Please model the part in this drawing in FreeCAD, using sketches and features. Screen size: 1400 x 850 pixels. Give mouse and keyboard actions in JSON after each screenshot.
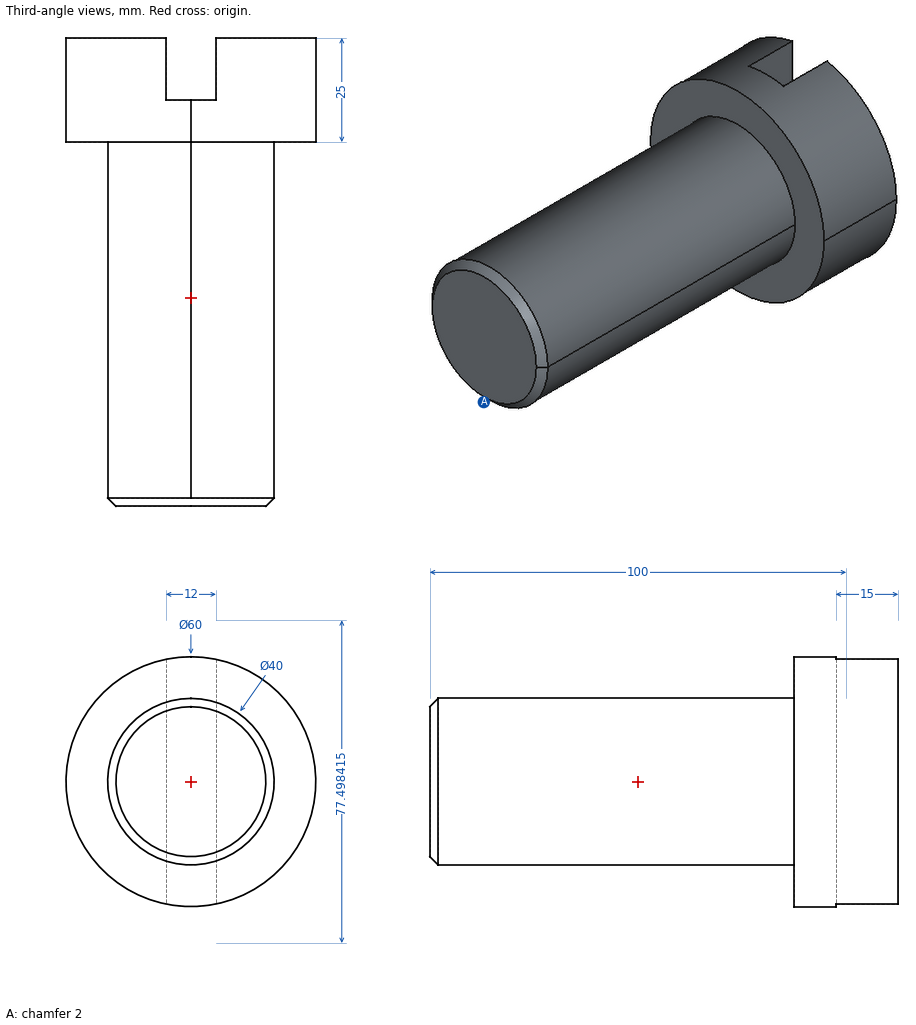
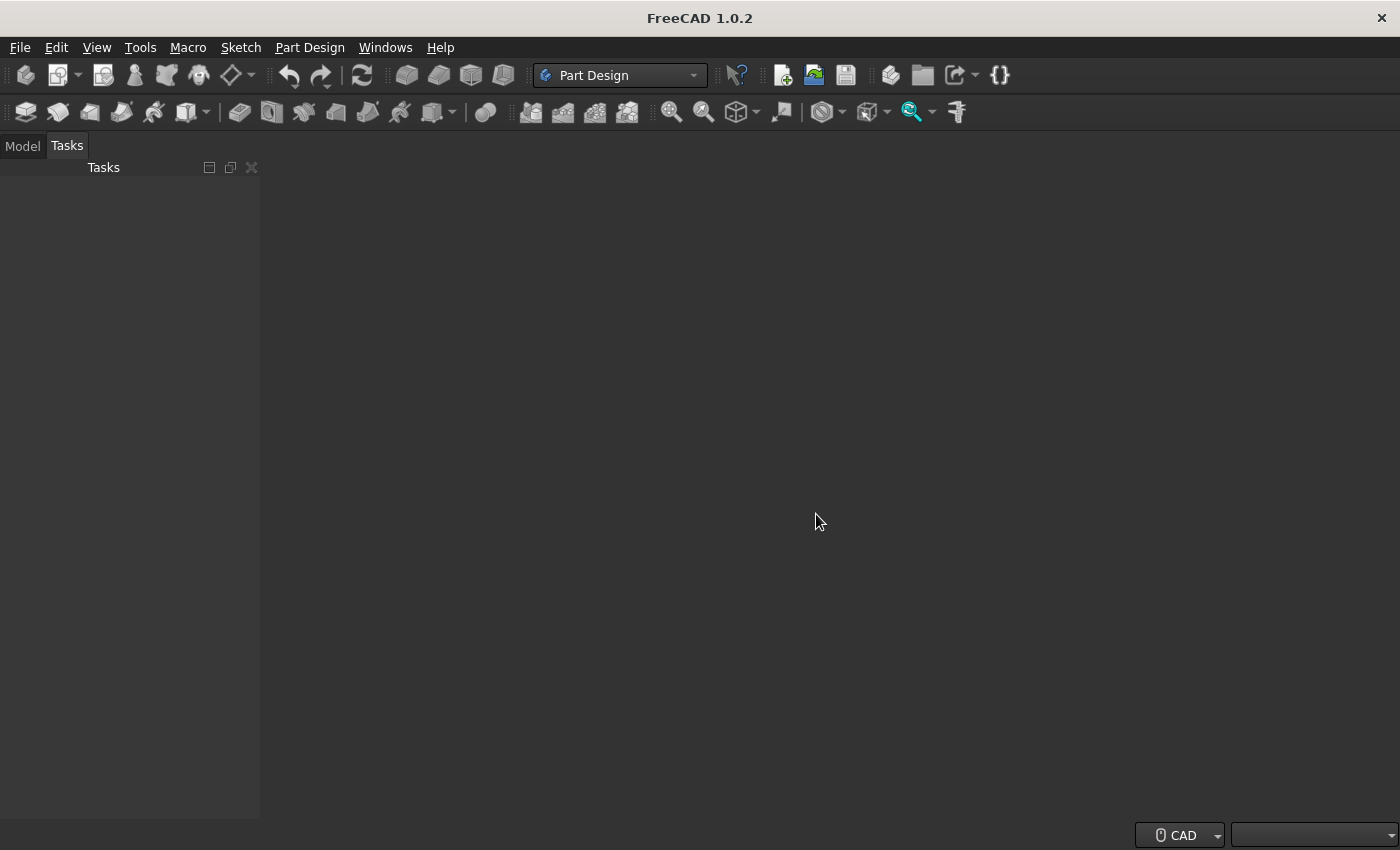
{"action": "left_click", "coordinate": [782, 76]}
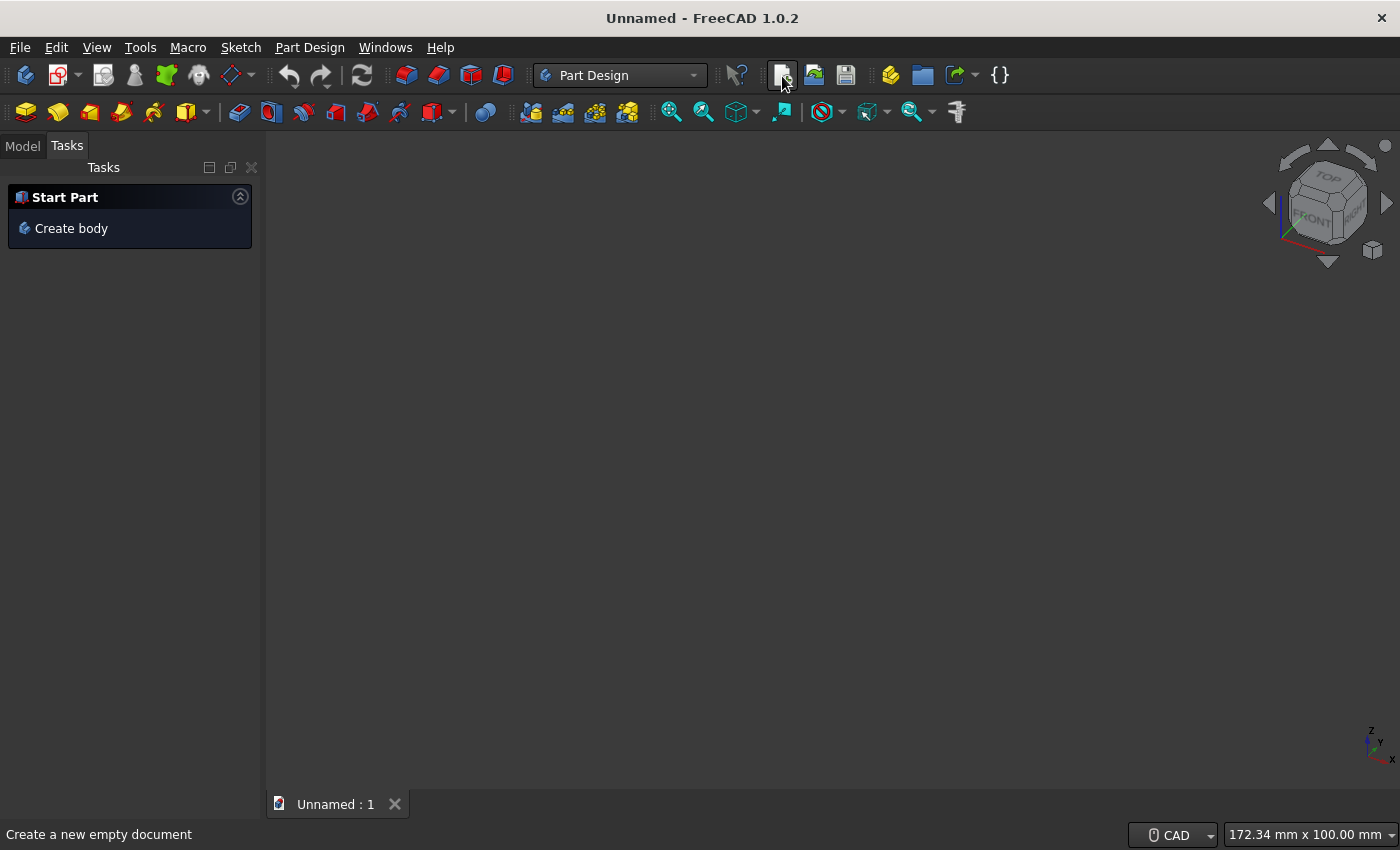
{"action": "left_click", "coordinate": [58, 76]}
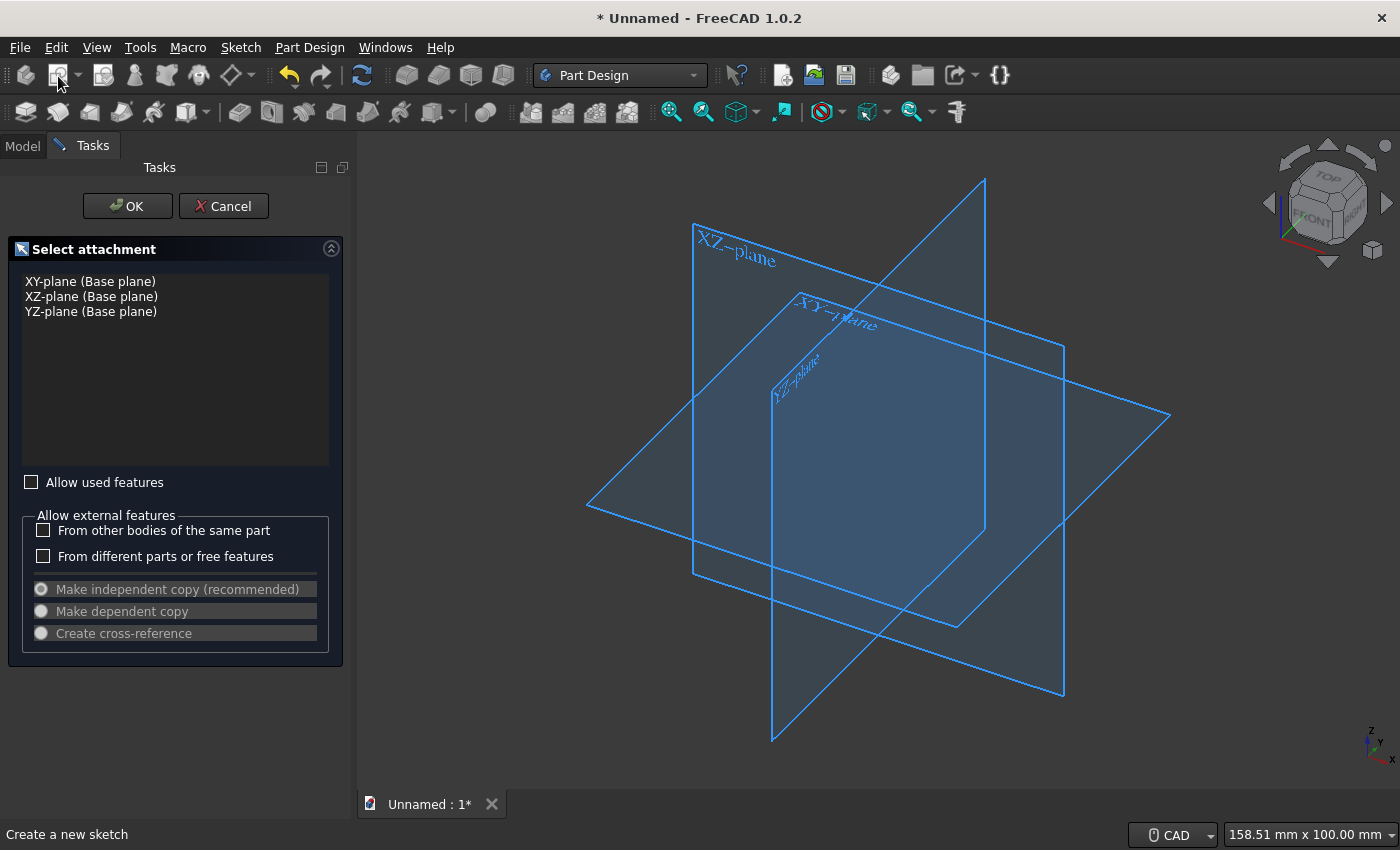
{"action": "left_click", "coordinate": [82, 296]}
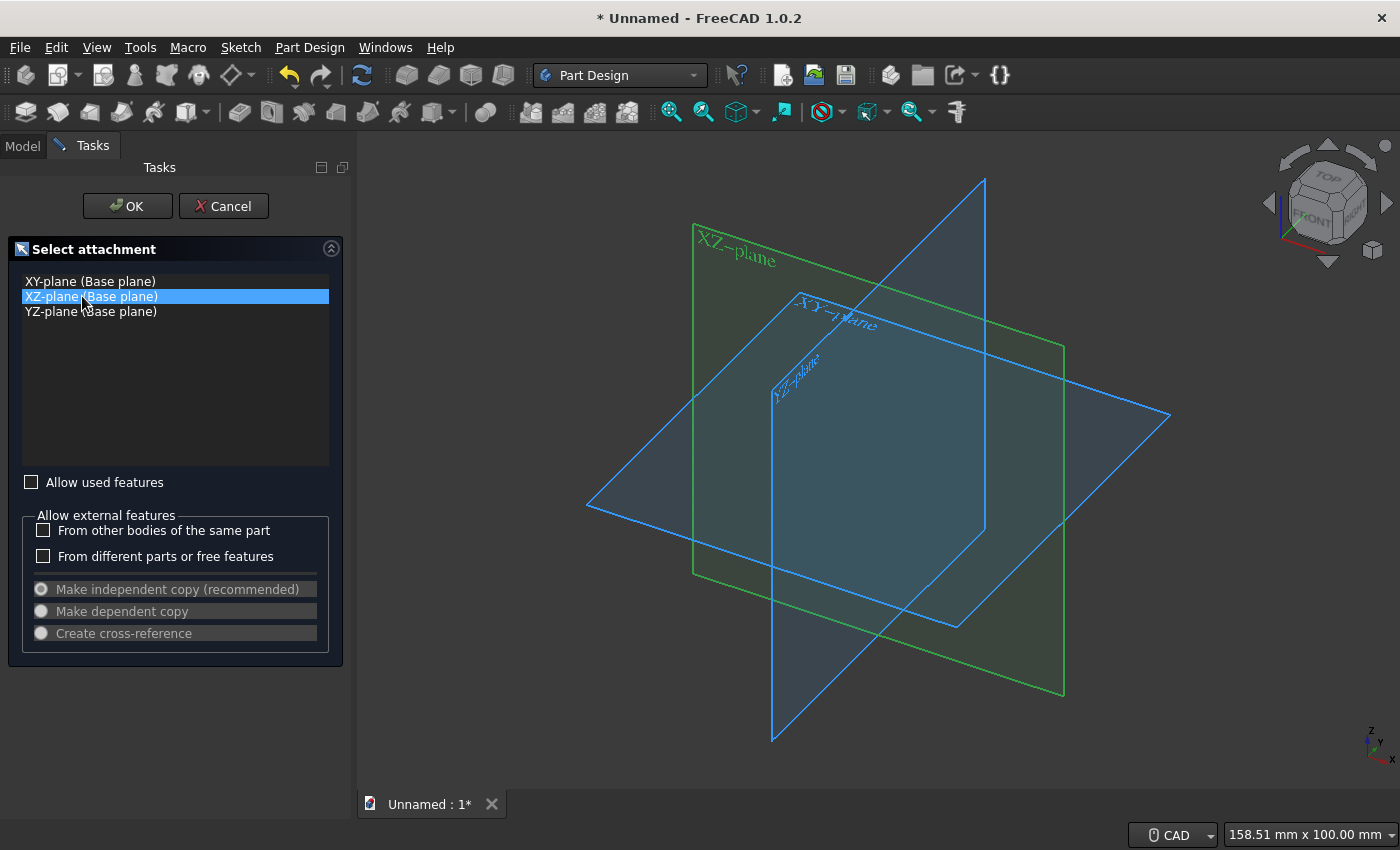
{"action": "left_click", "coordinate": [128, 206]}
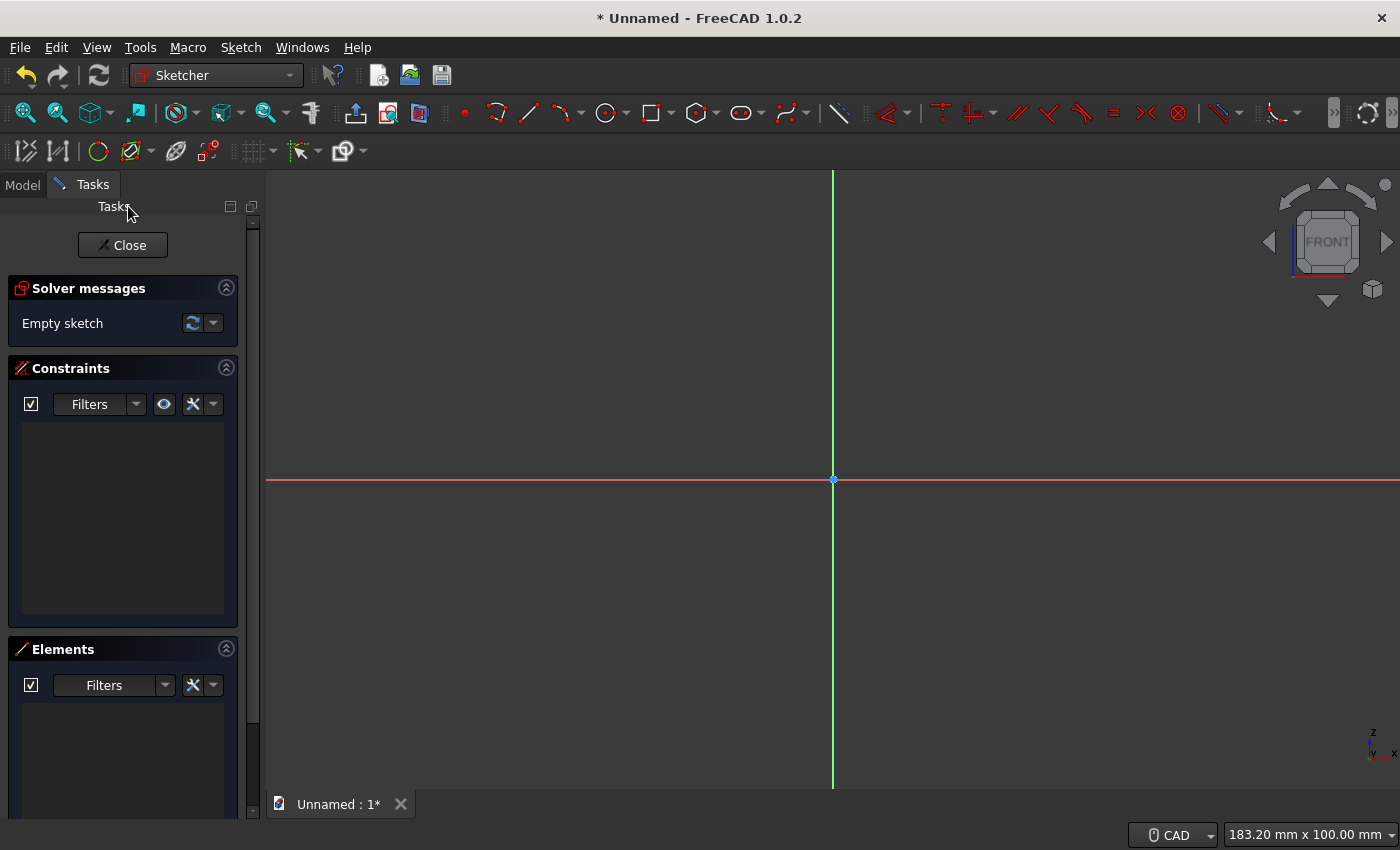
{"action": "scroll", "coordinate": [972, 480], "scroll_direction": "up", "scroll_amount": 2}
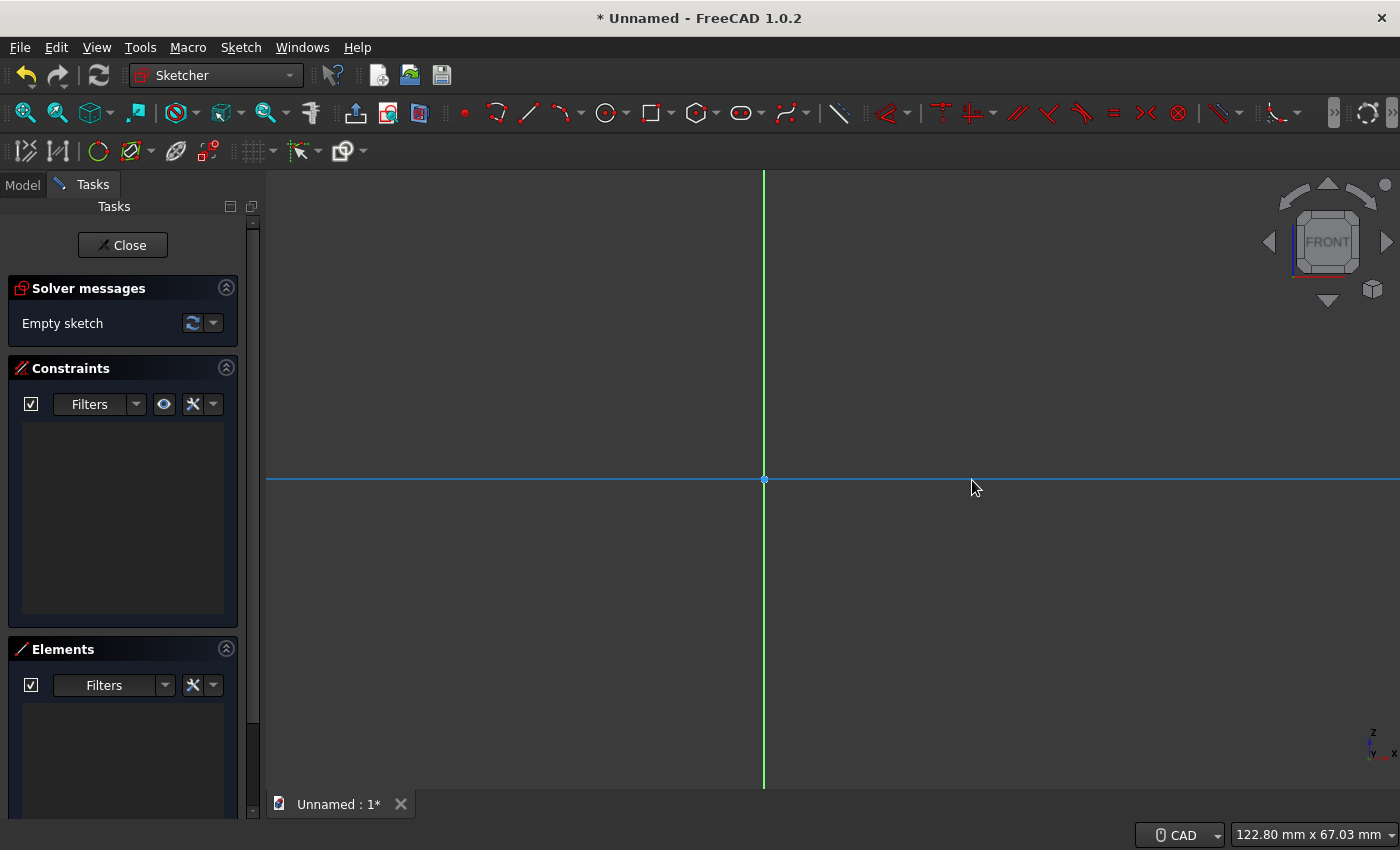
{"action": "left_click", "coordinate": [606, 114]}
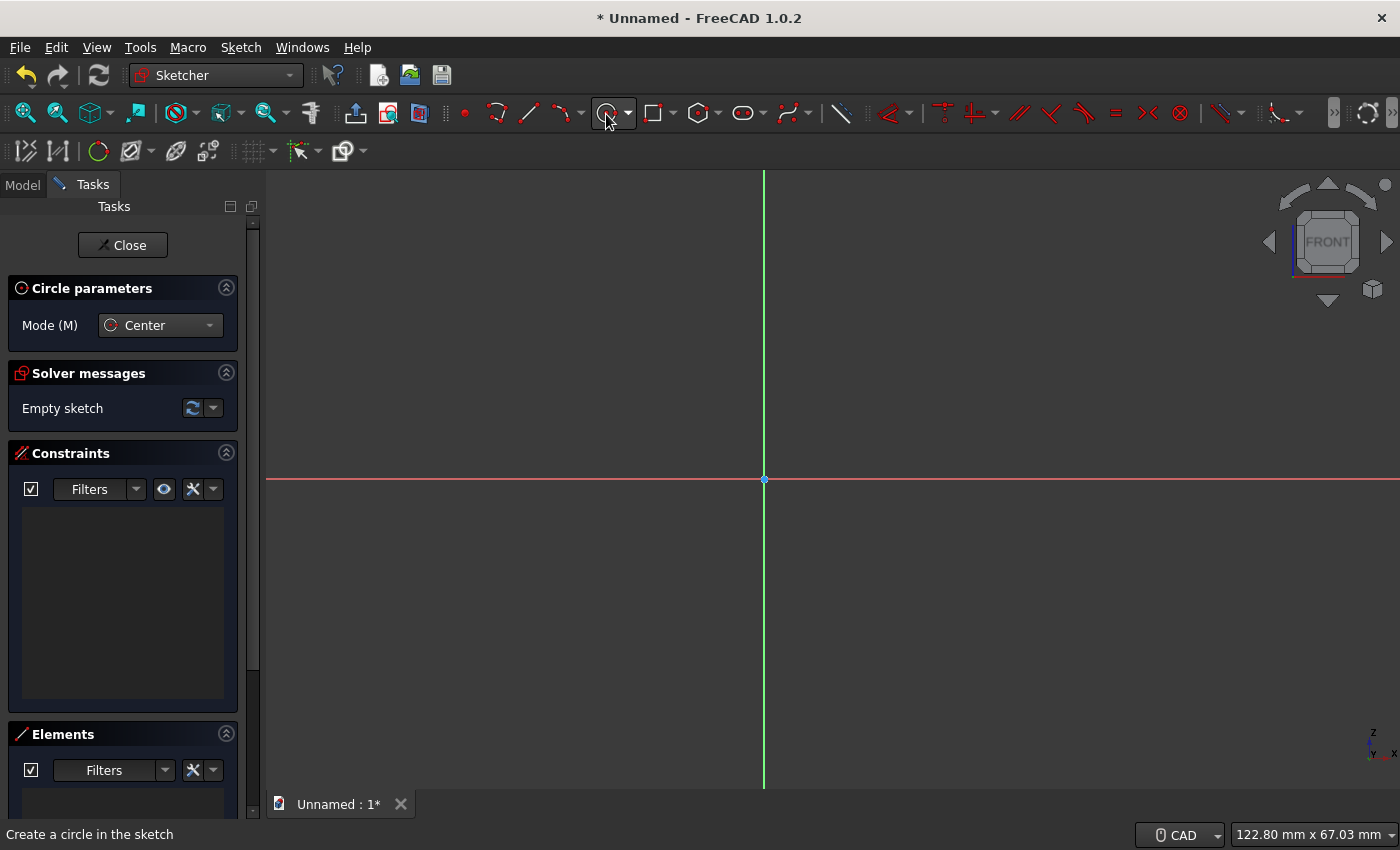
{"action": "left_click", "coordinate": [764, 479]}
{"action": "mouse_move", "coordinate": [895, 348]}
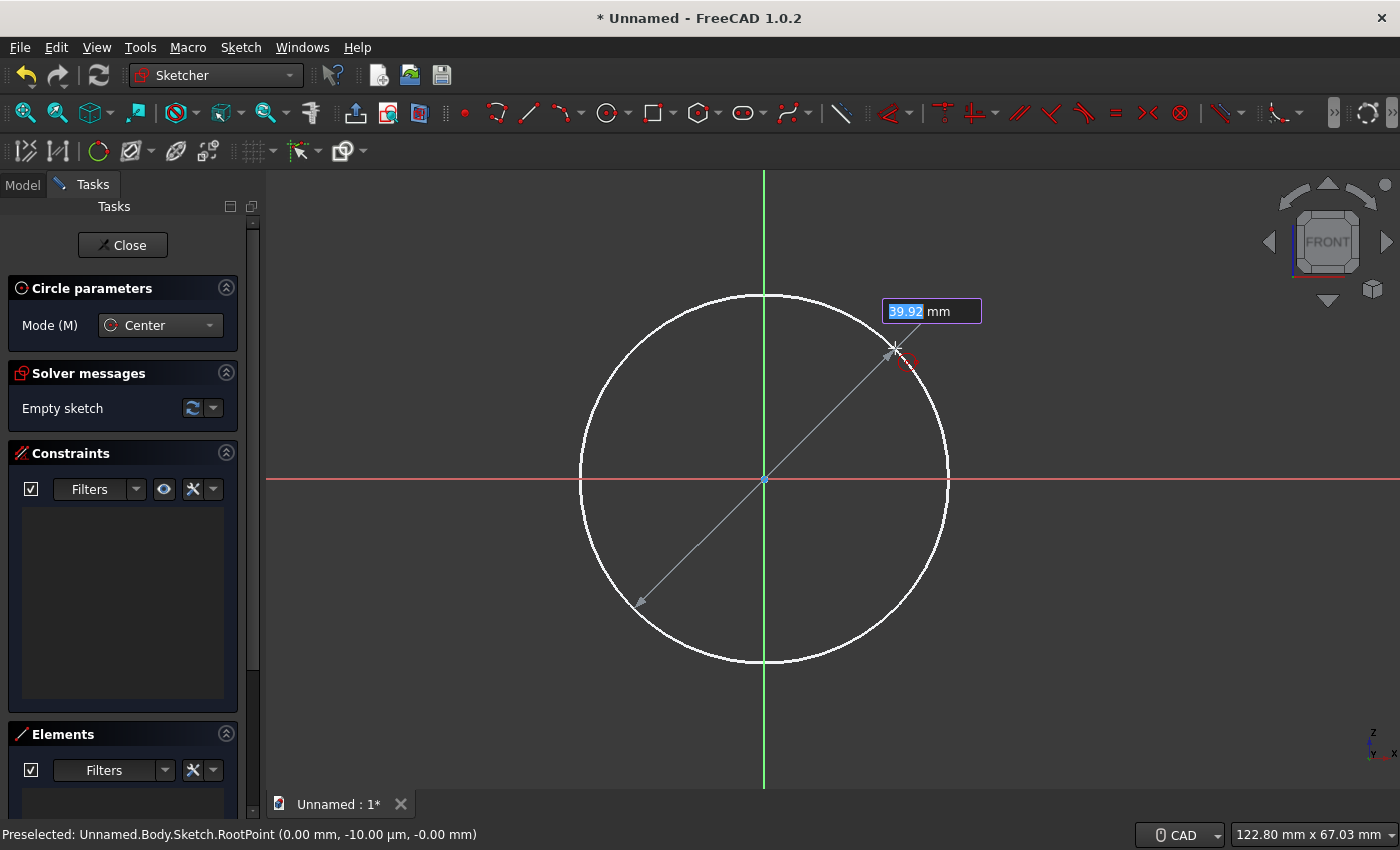
{"action": "type", "text": "40"}
{"action": "key", "text": "Return"}
{"action": "key", "text": "Escape"}